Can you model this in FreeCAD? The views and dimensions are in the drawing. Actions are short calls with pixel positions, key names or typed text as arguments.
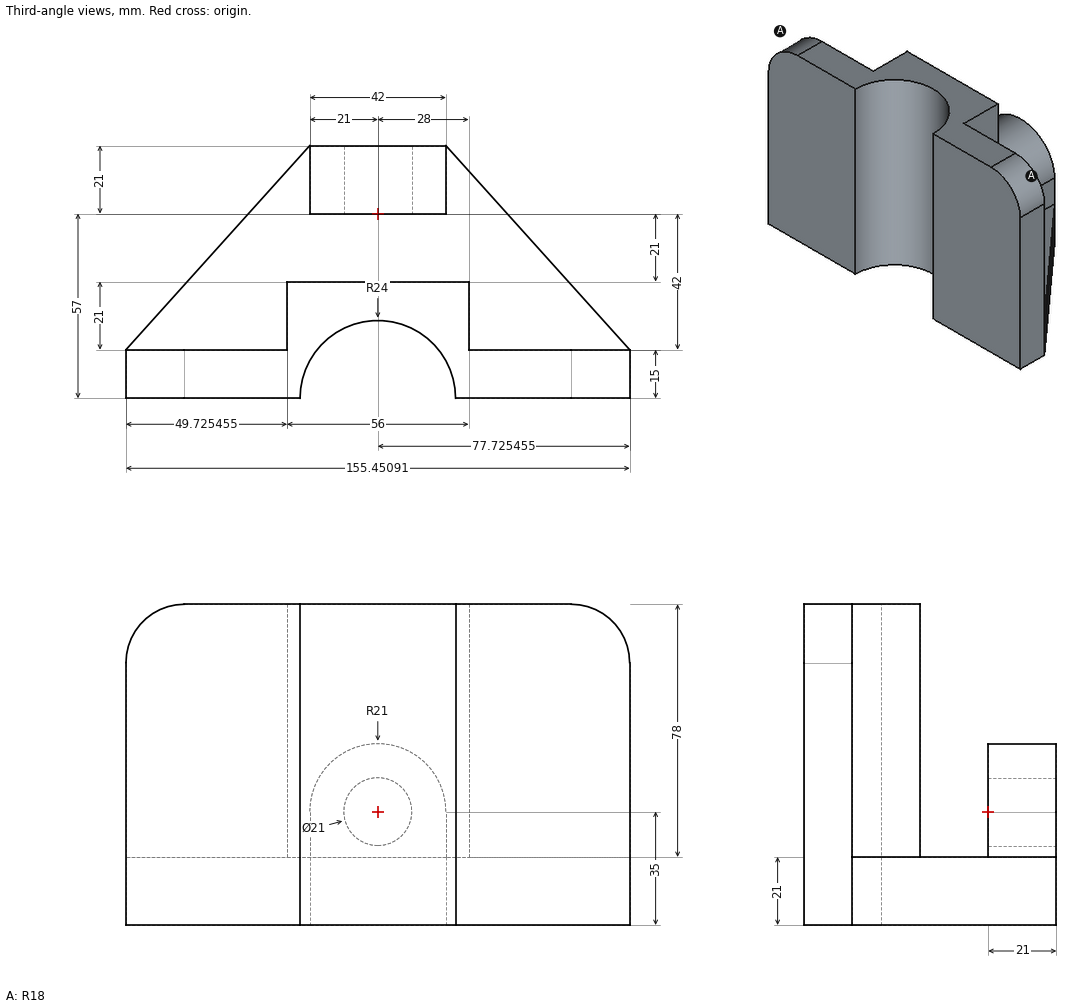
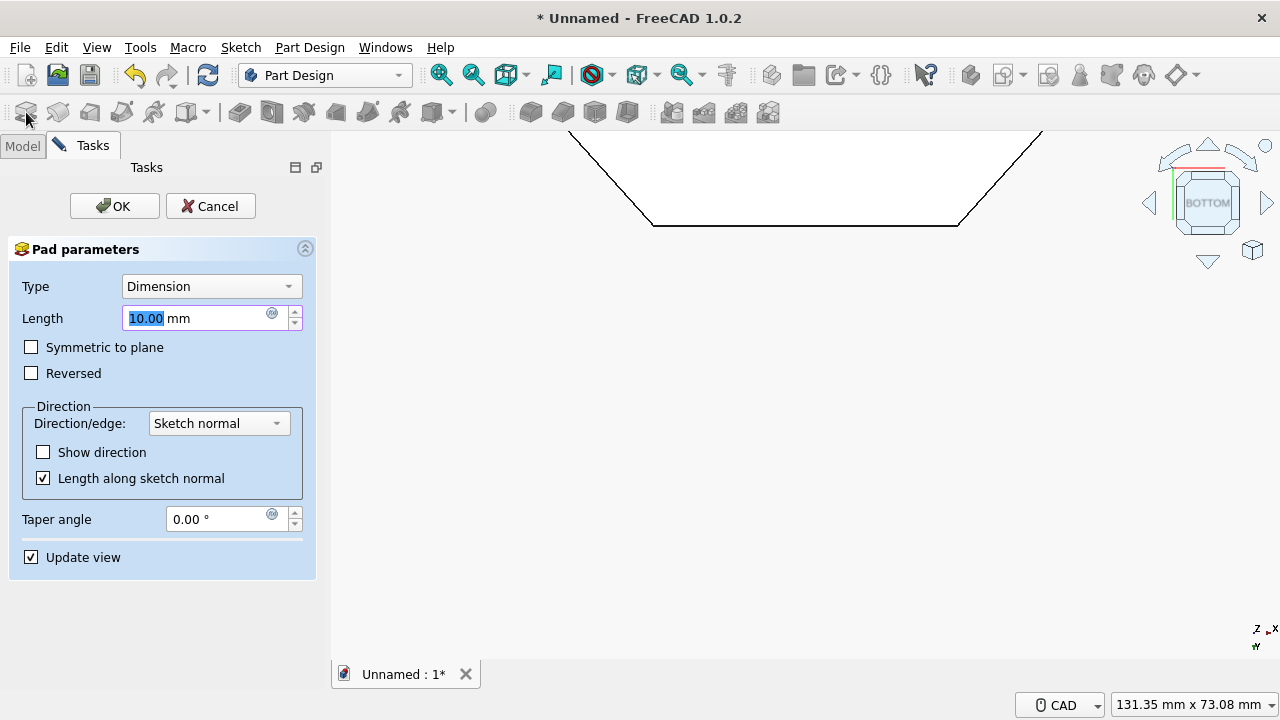
text(21)
key(Tab)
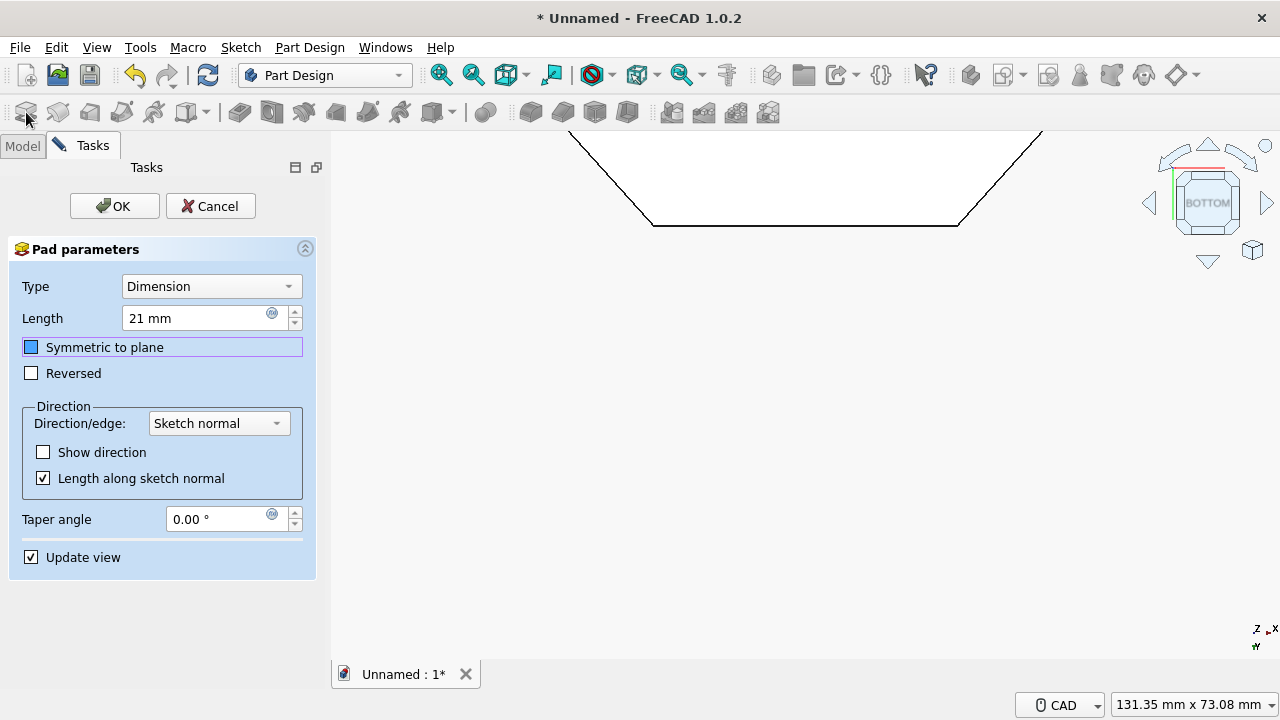
click(30, 373)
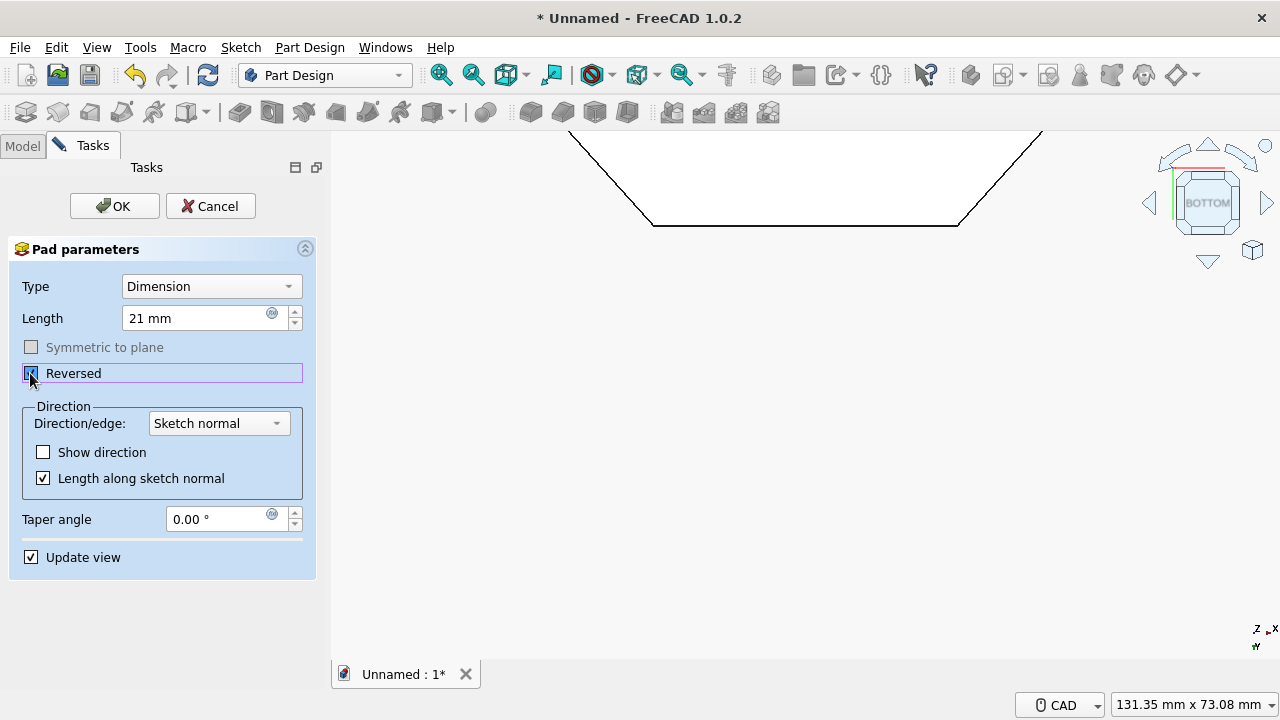
click(115, 206)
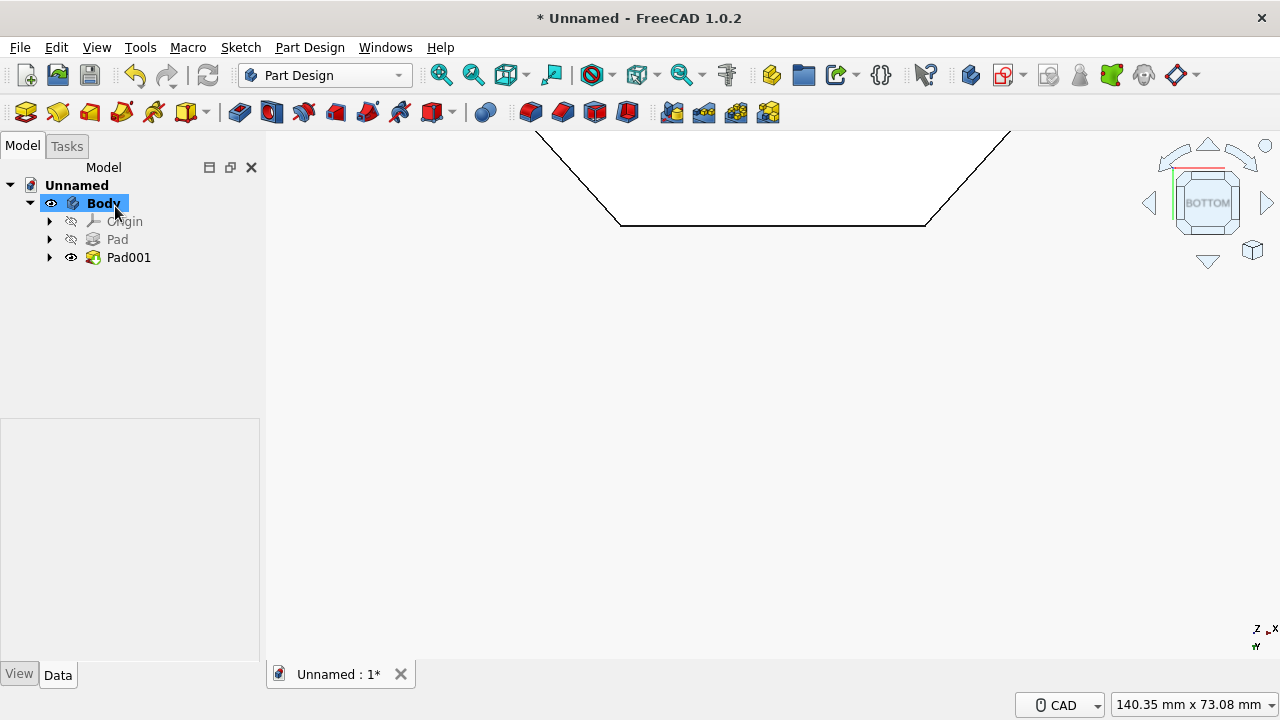
click(442, 76)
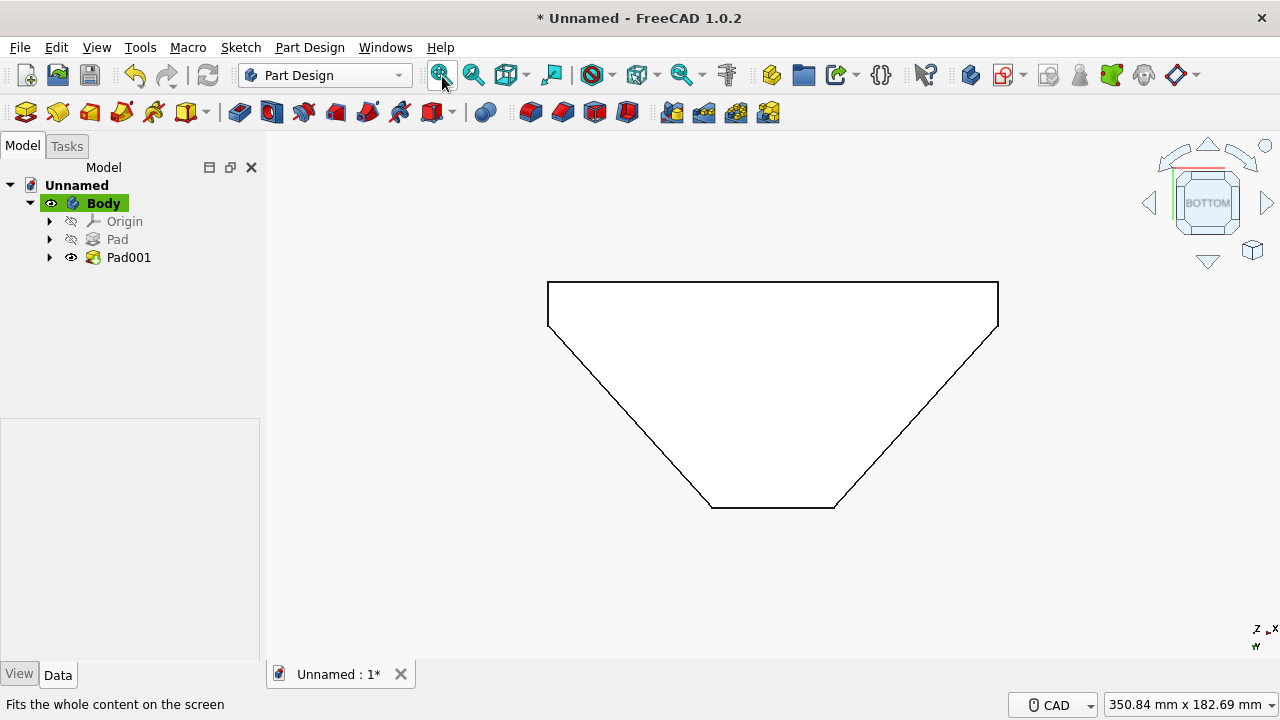
key(0)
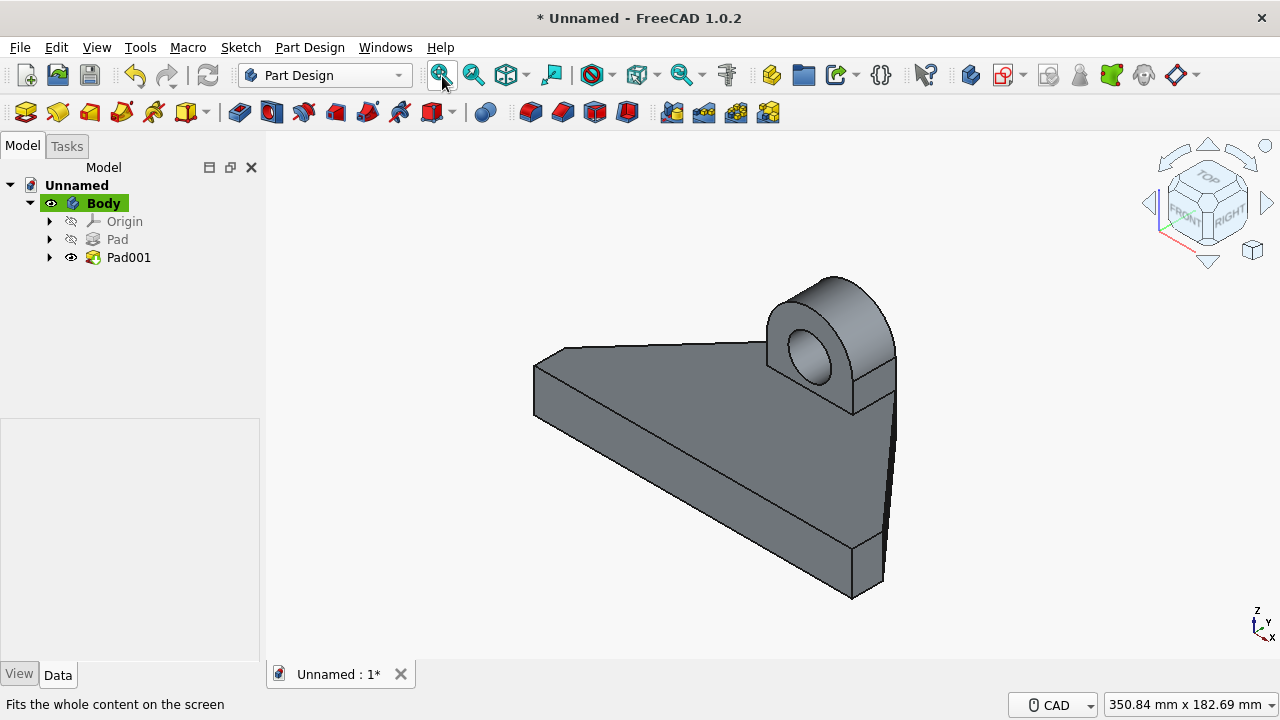
click(796, 450)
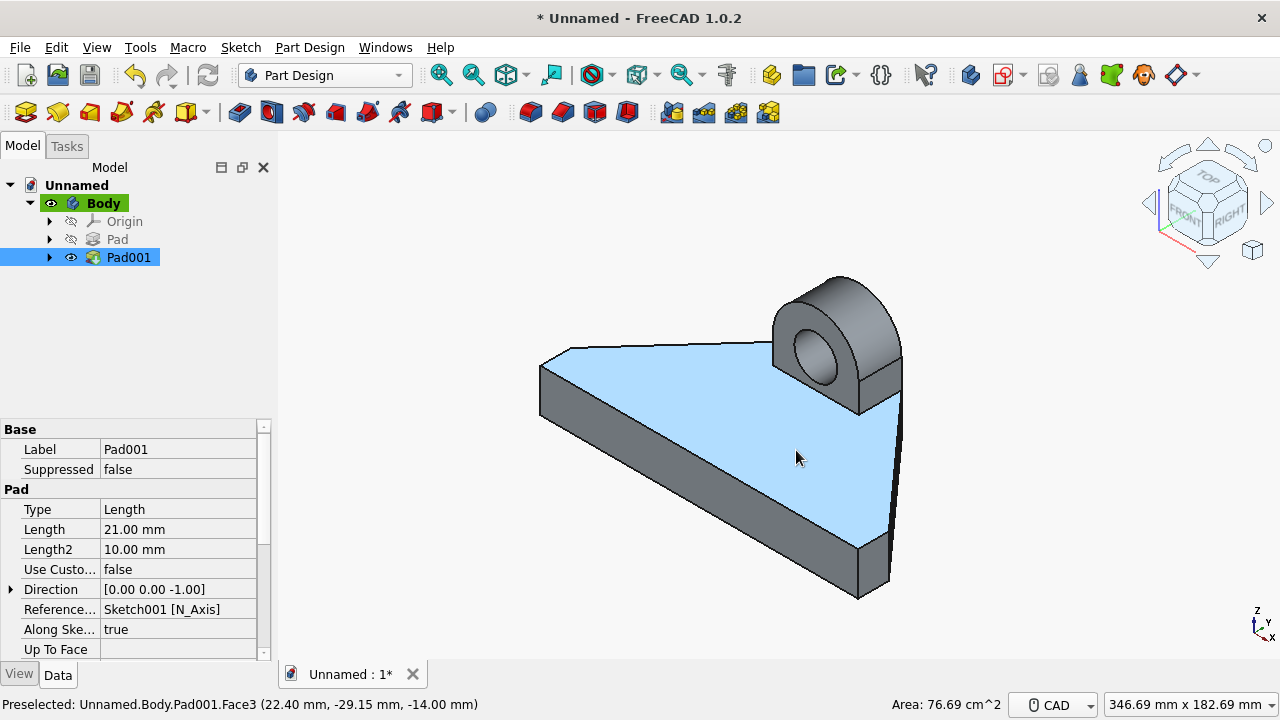
click(1004, 76)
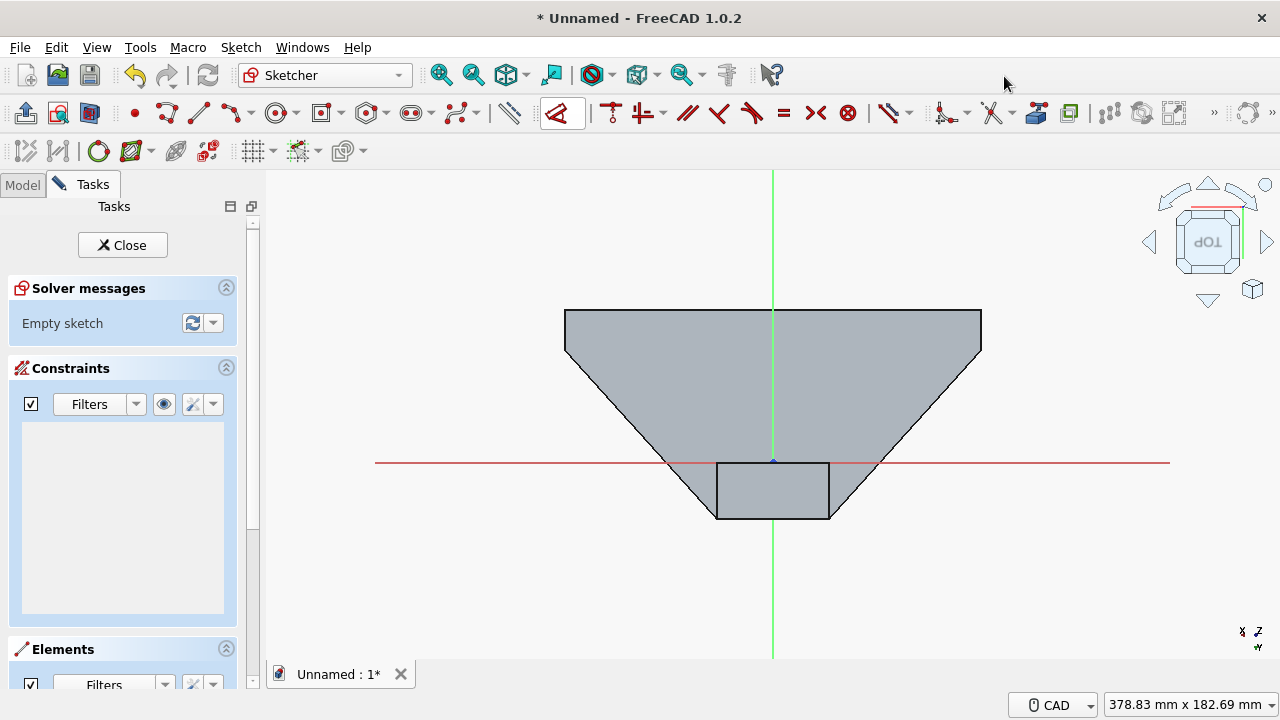
scroll(912, 329, up, 2)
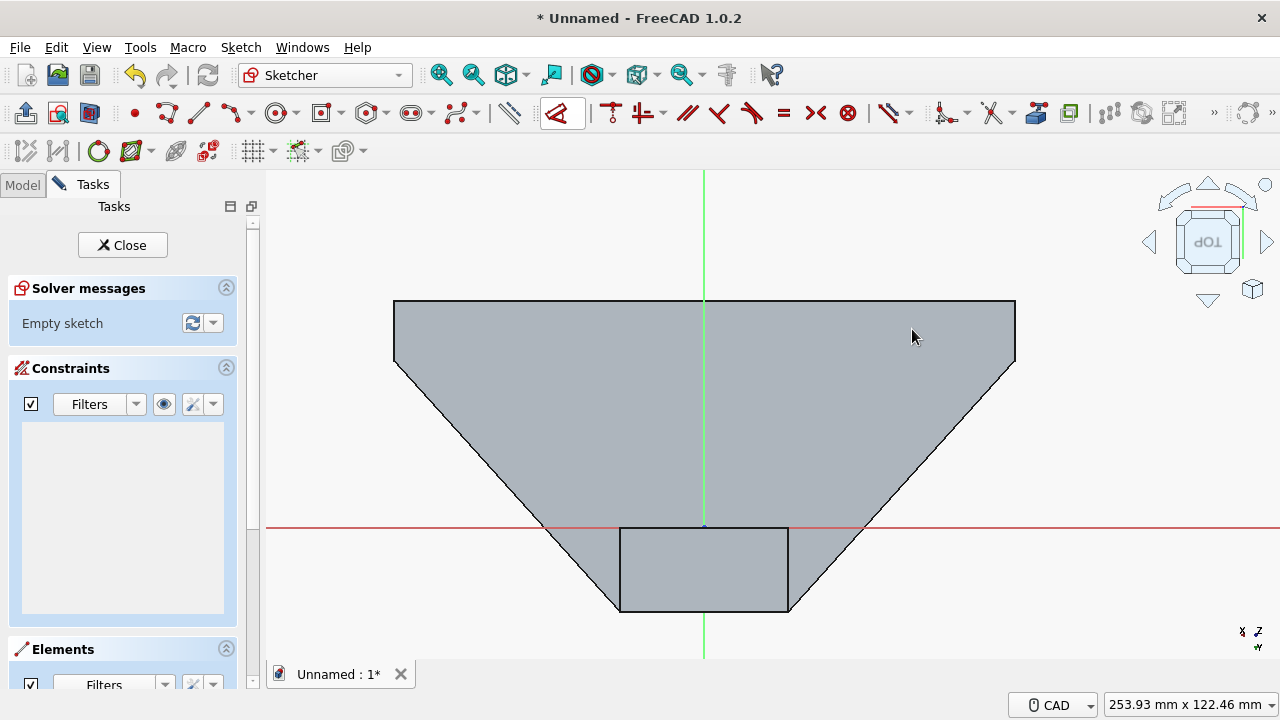
click(168, 114)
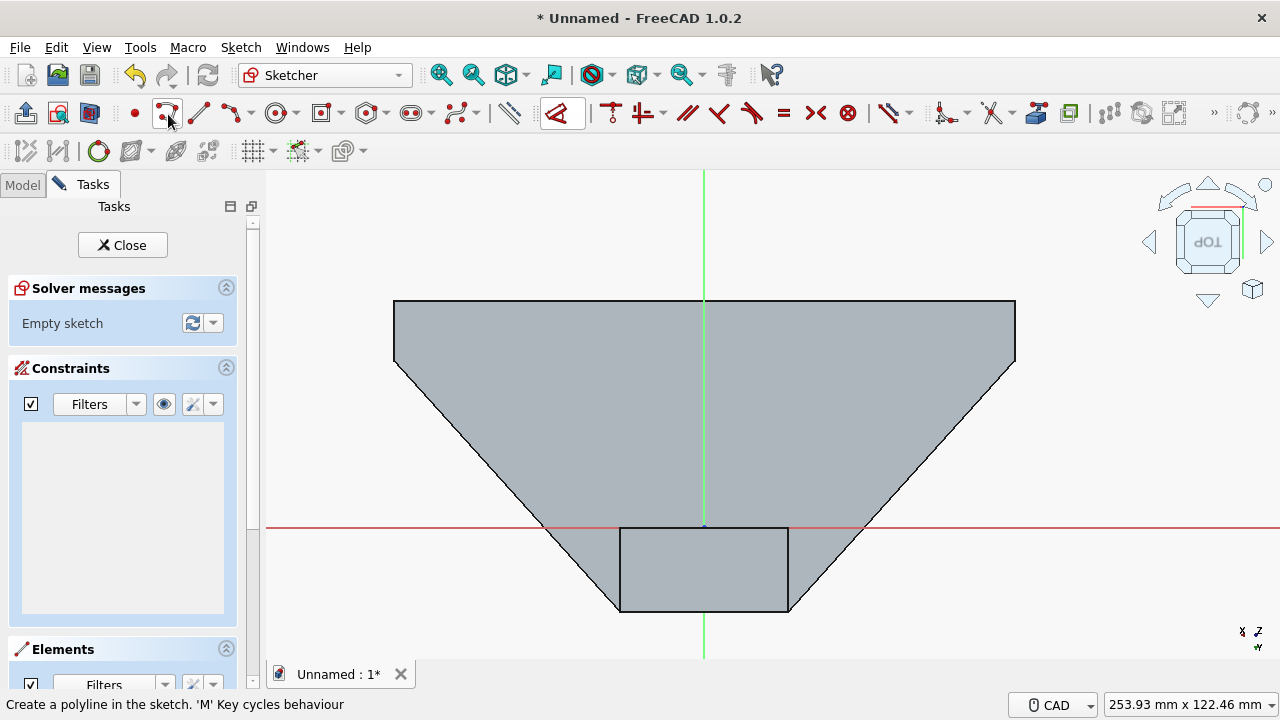
click(593, 444)
click(816, 444)
click(816, 361)
click(1015, 361)
click(1015, 301)
click(394, 301)
click(394, 361)
click(593, 361)
click(593, 445)
key(Escape)
key(Escape)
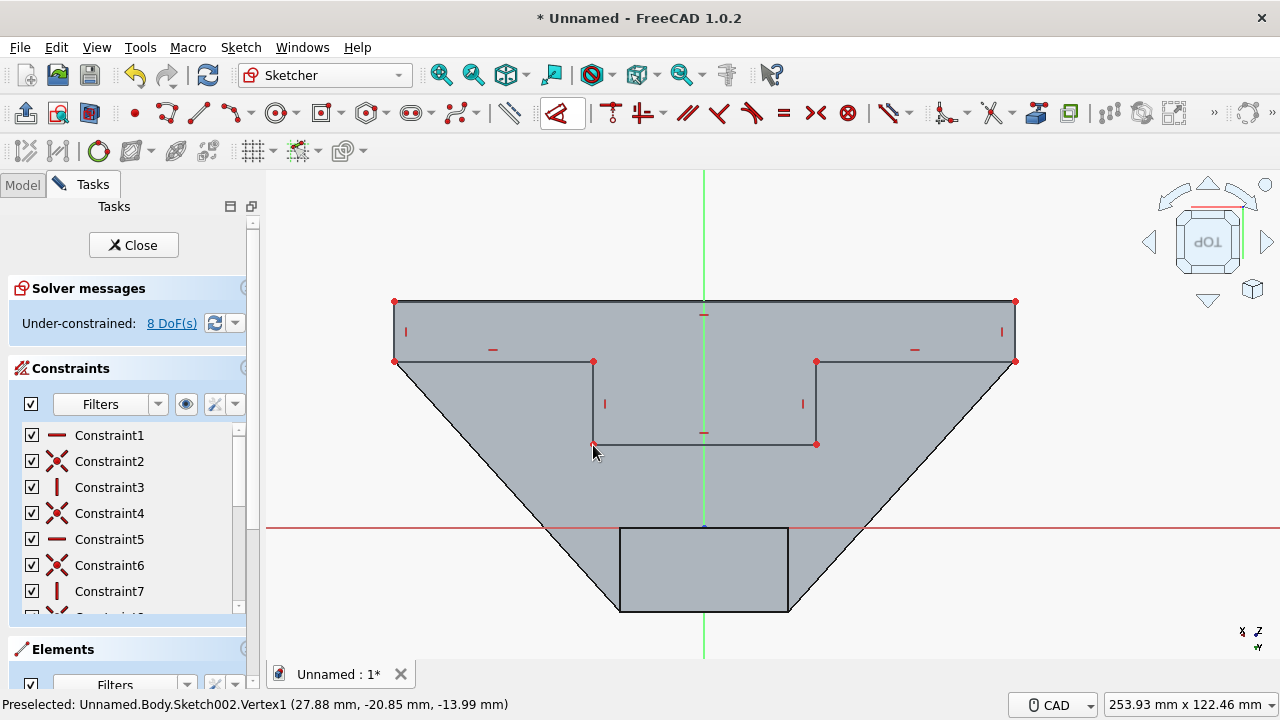
click(660, 445)